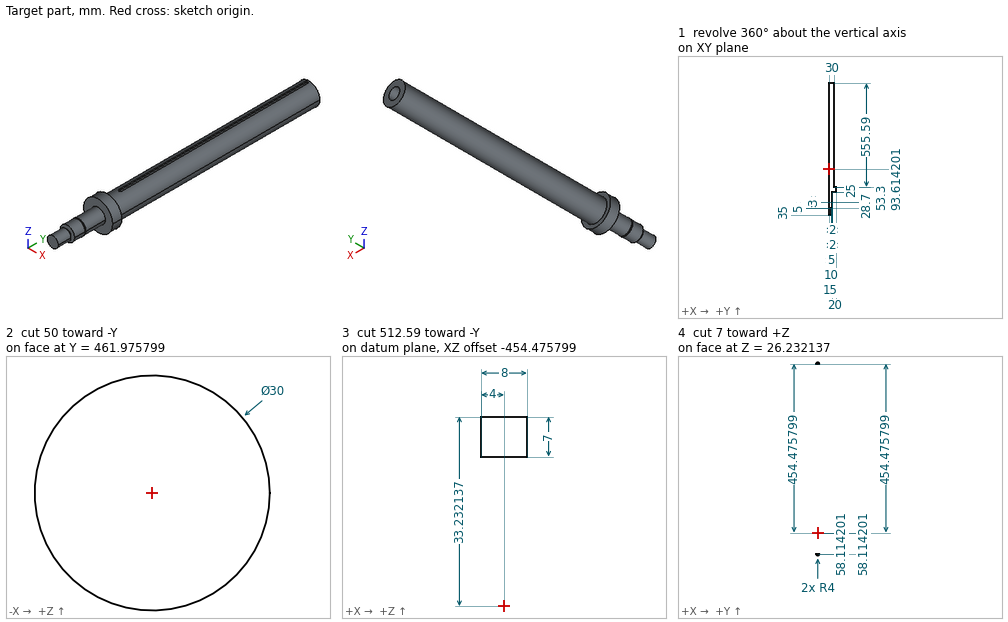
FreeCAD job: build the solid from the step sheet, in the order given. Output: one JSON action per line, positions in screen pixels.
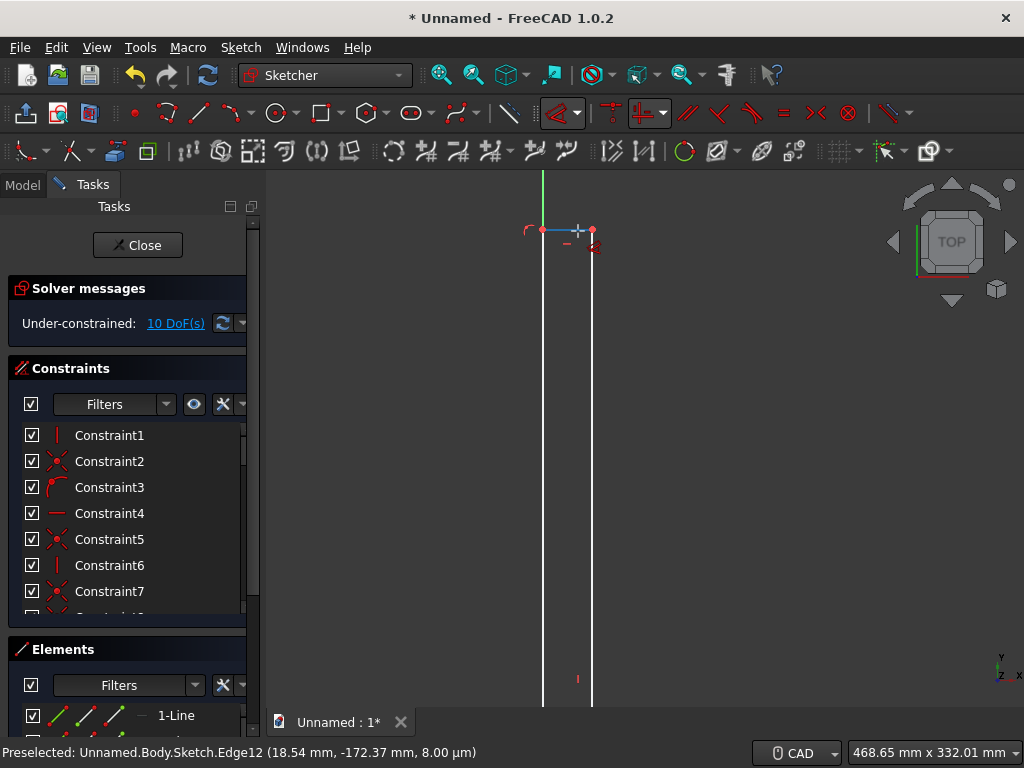
{"action": "left_click", "coordinate": [577, 230]}
{"action": "left_click", "coordinate": [567, 264]}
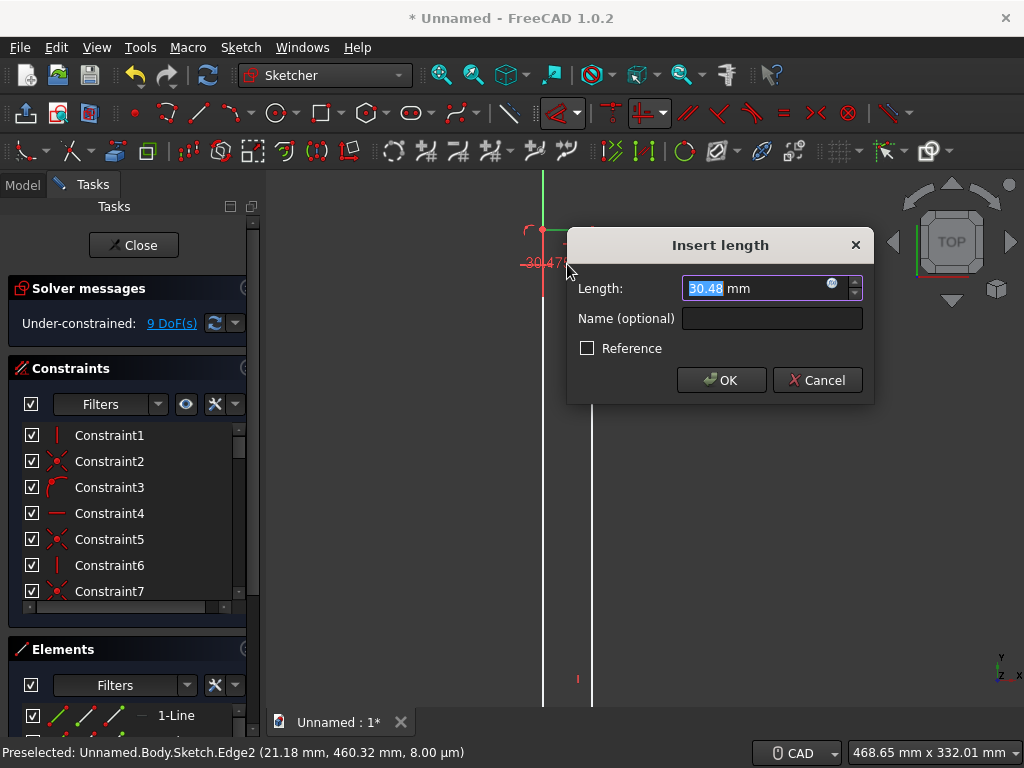
{"action": "type", "text": "30"}
{"action": "key", "text": "Return"}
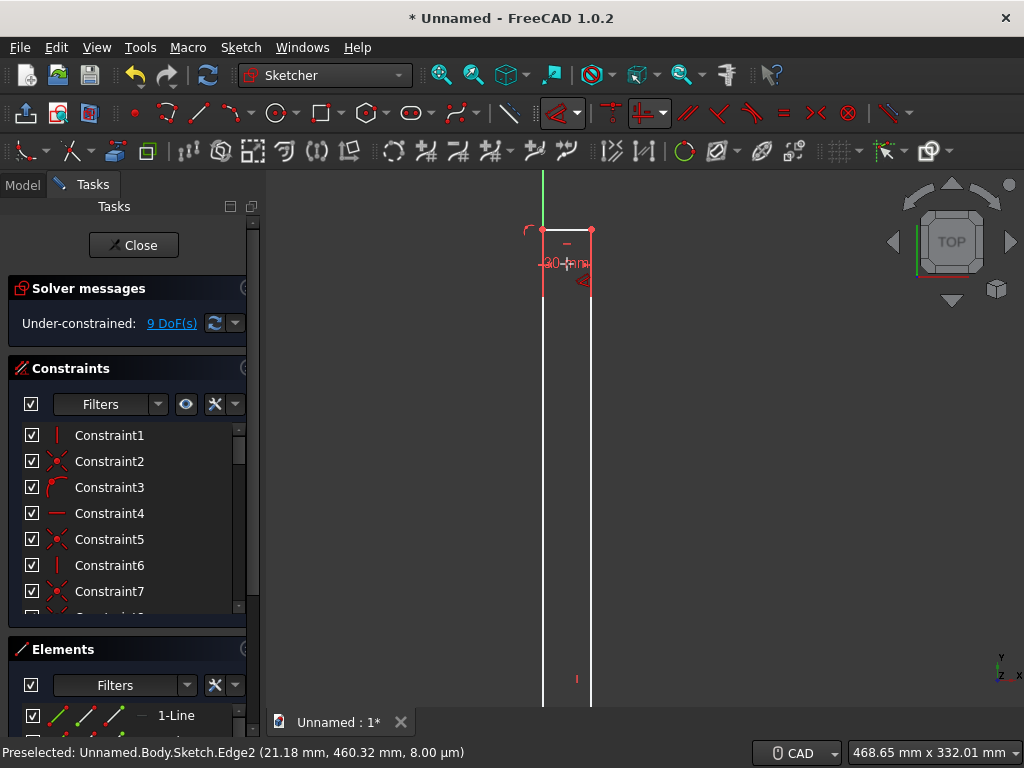
{"action": "scroll", "coordinate": [577, 284], "scroll_direction": "down", "scroll_amount": 6}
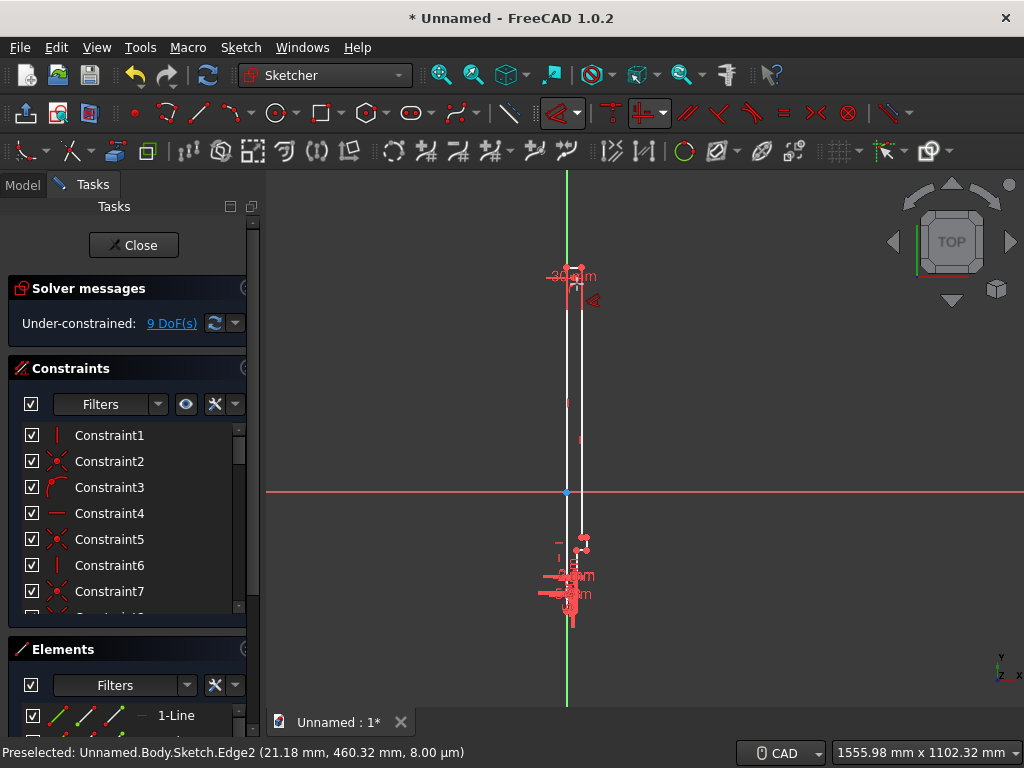
{"action": "scroll", "coordinate": [570, 612], "scroll_direction": "up", "scroll_amount": 9}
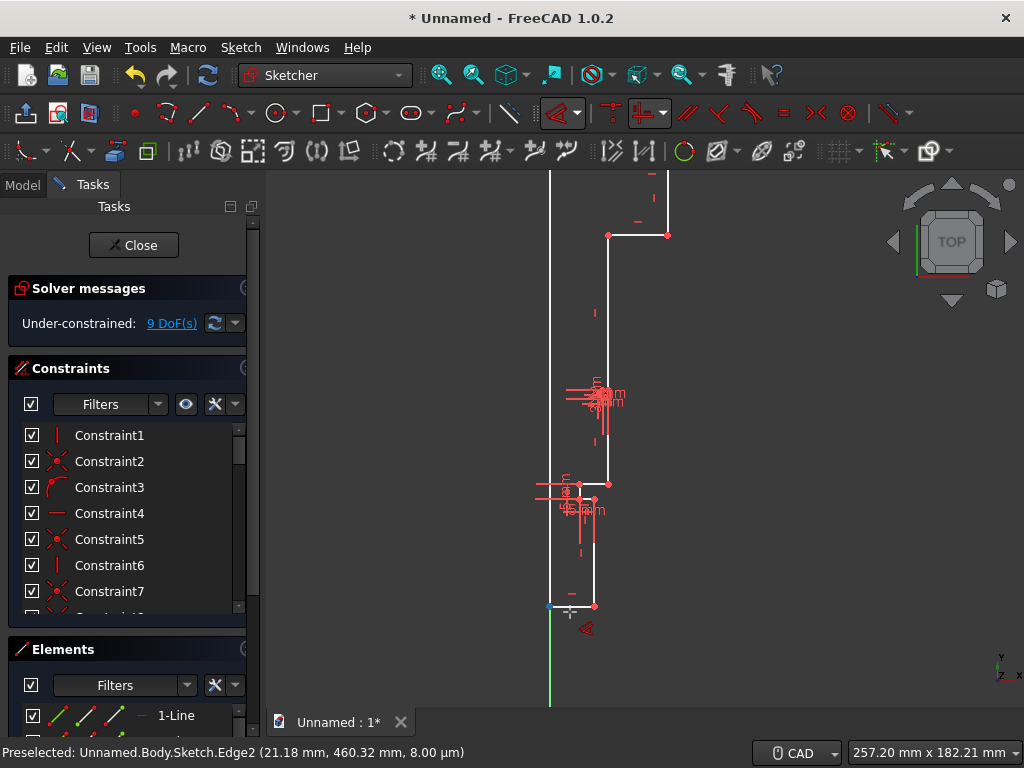
{"action": "left_click", "coordinate": [568, 607]}
{"action": "left_click", "coordinate": [572, 641]}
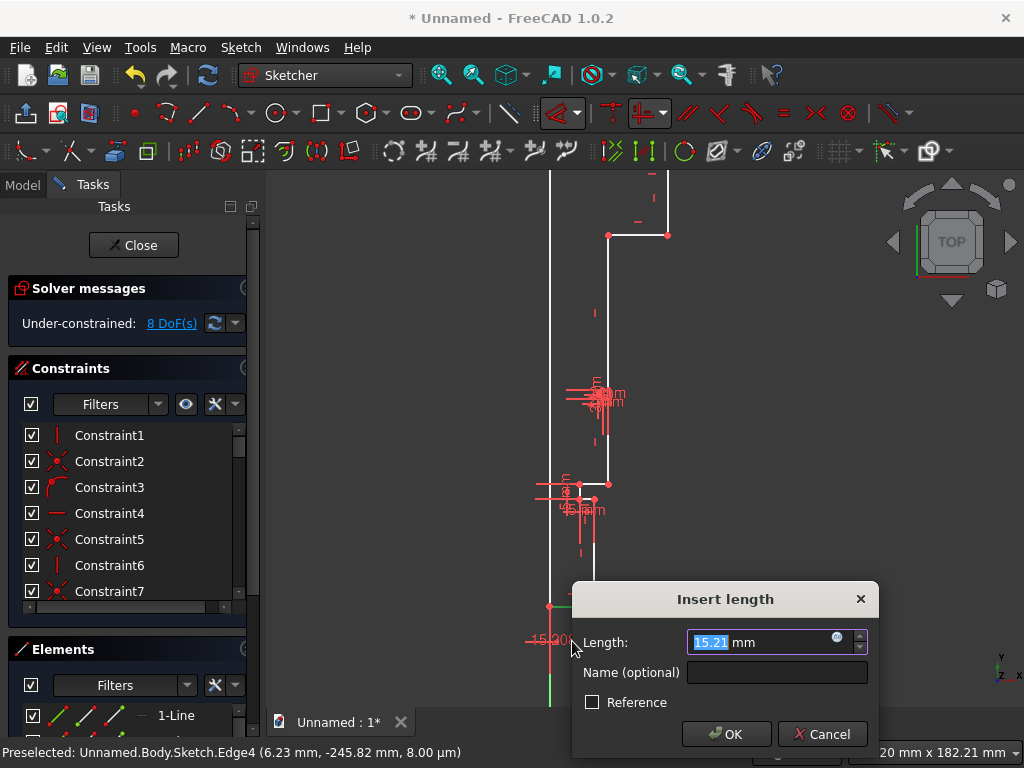
{"action": "type", "text": "15"}
{"action": "key", "text": "Return"}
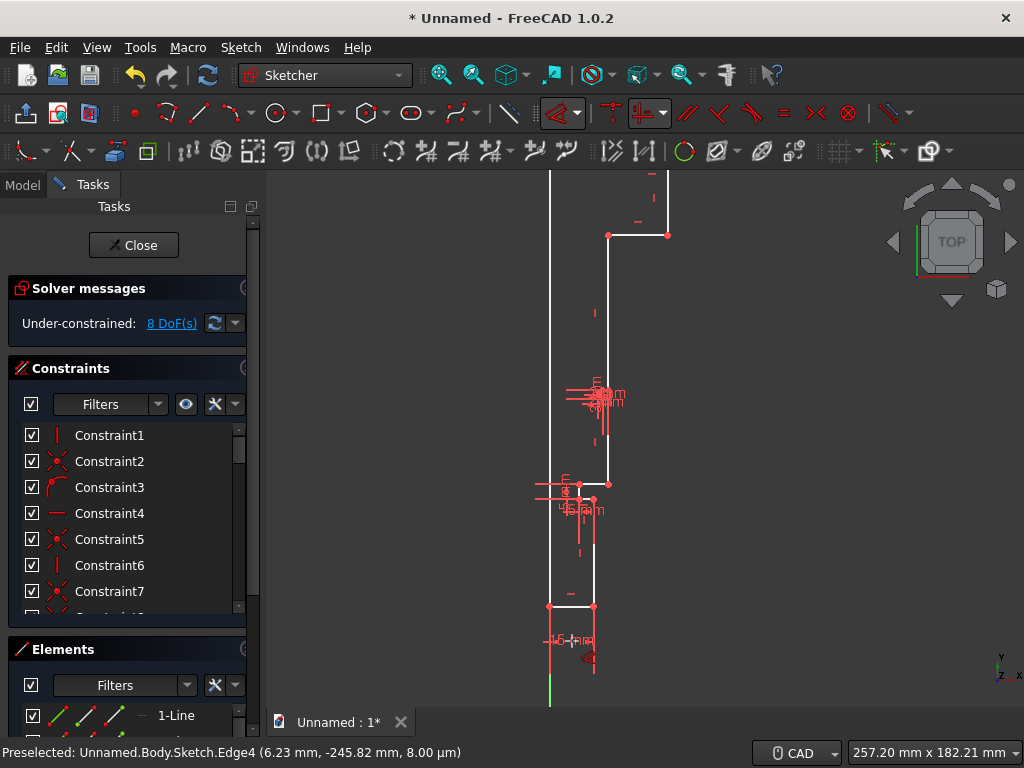
{"action": "left_click", "coordinate": [594, 574]}
{"action": "left_click", "coordinate": [628, 553]}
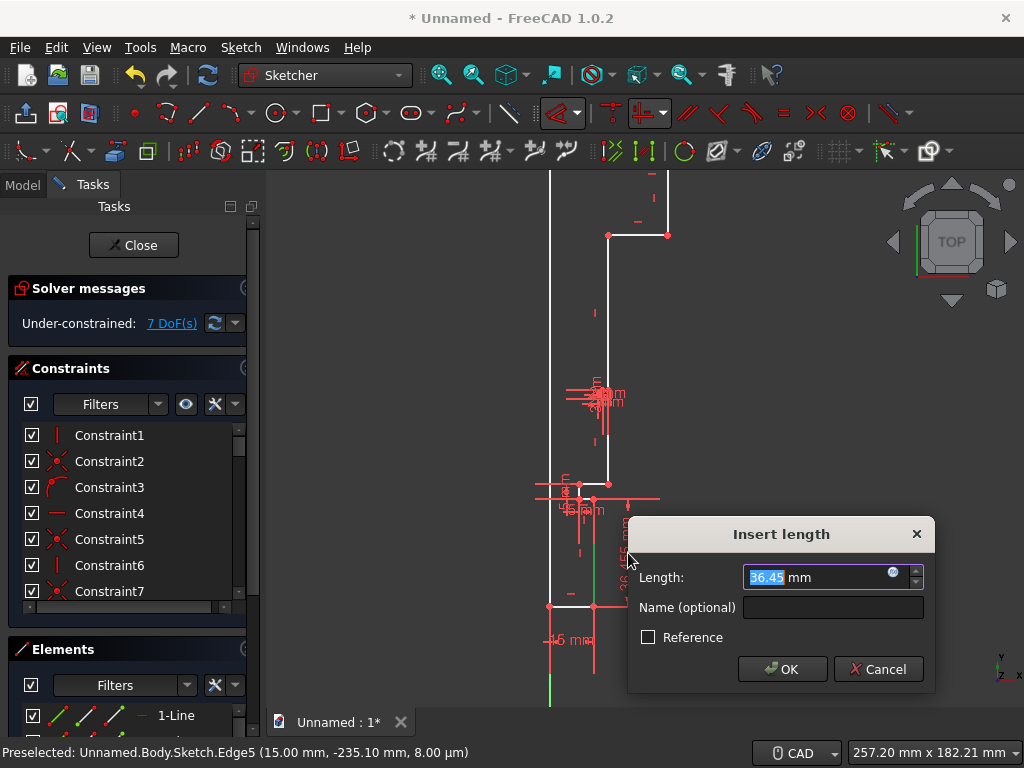
{"action": "type", "text": "35"}
{"action": "key", "text": "Return"}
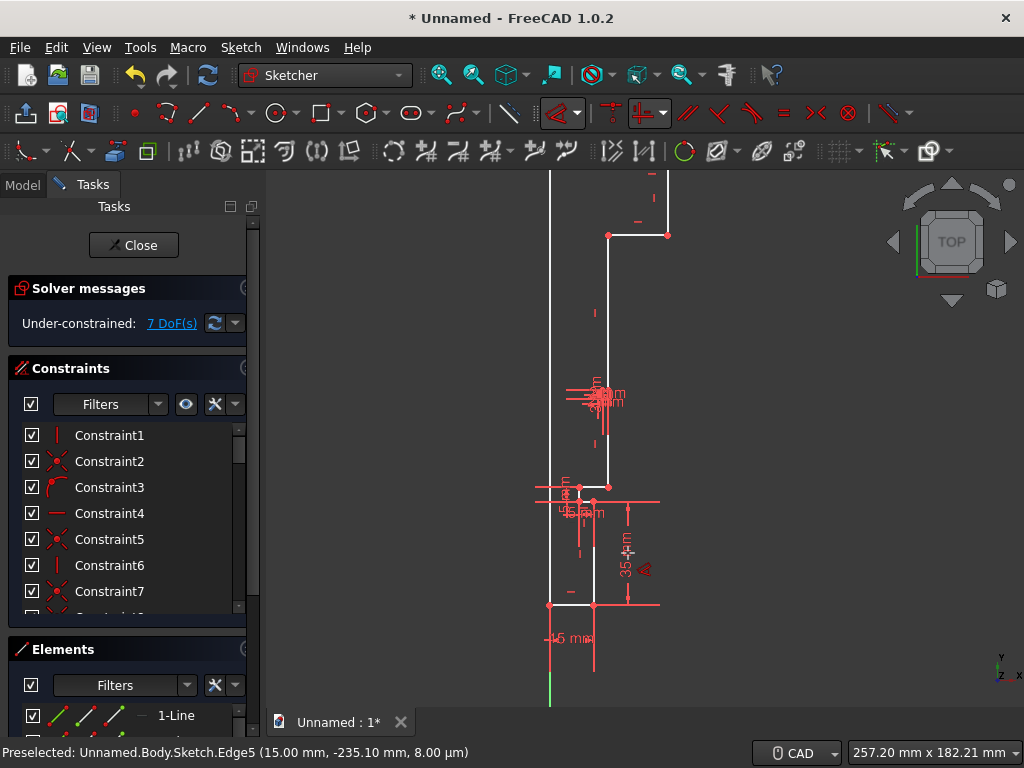
{"action": "scroll", "coordinate": [591, 487], "scroll_direction": "up", "scroll_amount": 2}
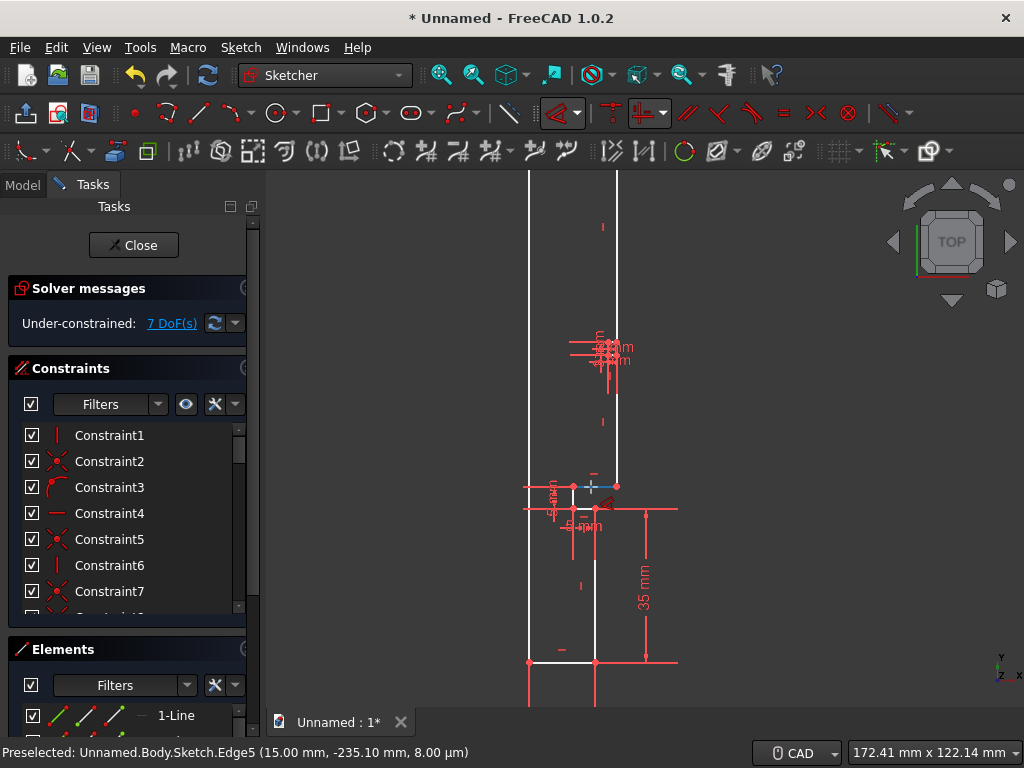
{"action": "left_click", "coordinate": [591, 487]}
{"action": "left_click", "coordinate": [595, 453]}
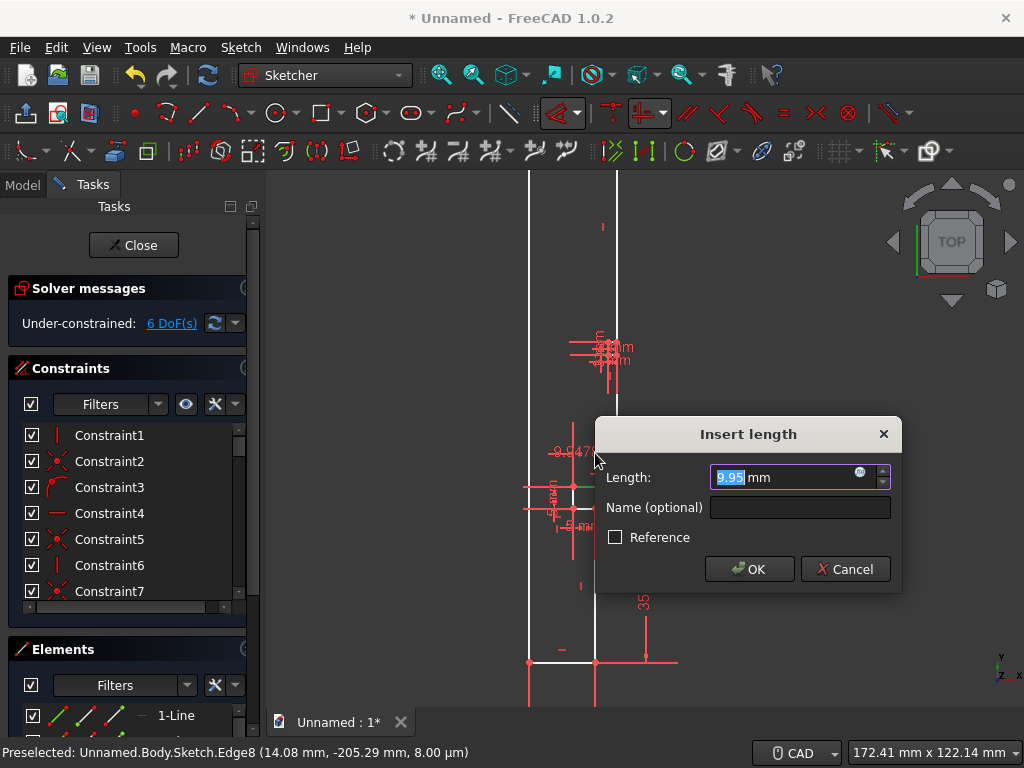
{"action": "type", "text": "10"}
{"action": "key", "text": "Return"}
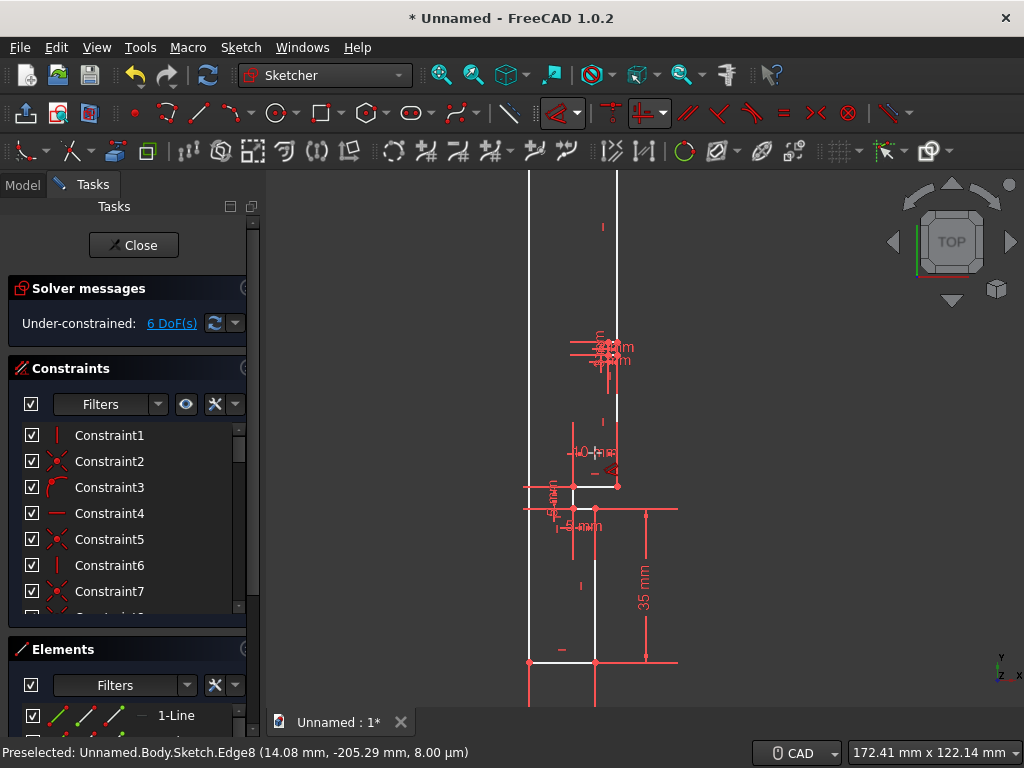
{"action": "scroll", "coordinate": [571, 605], "scroll_direction": "down", "scroll_amount": 11}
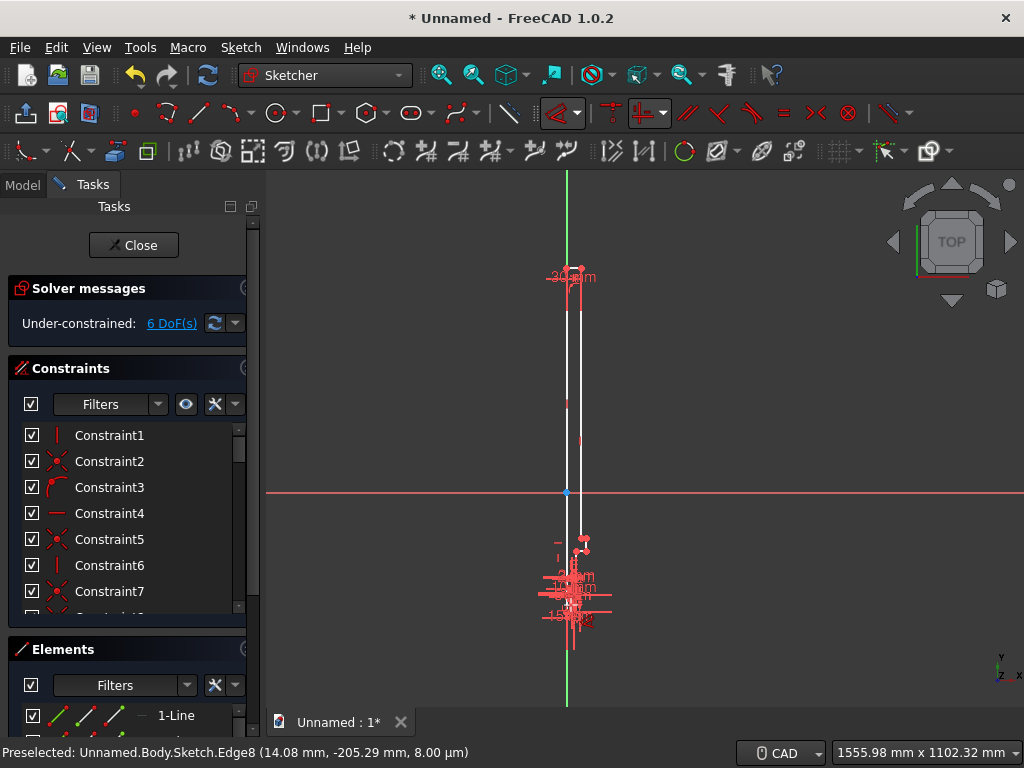
{"action": "scroll", "coordinate": [579, 551], "scroll_direction": "up", "scroll_amount": 8}